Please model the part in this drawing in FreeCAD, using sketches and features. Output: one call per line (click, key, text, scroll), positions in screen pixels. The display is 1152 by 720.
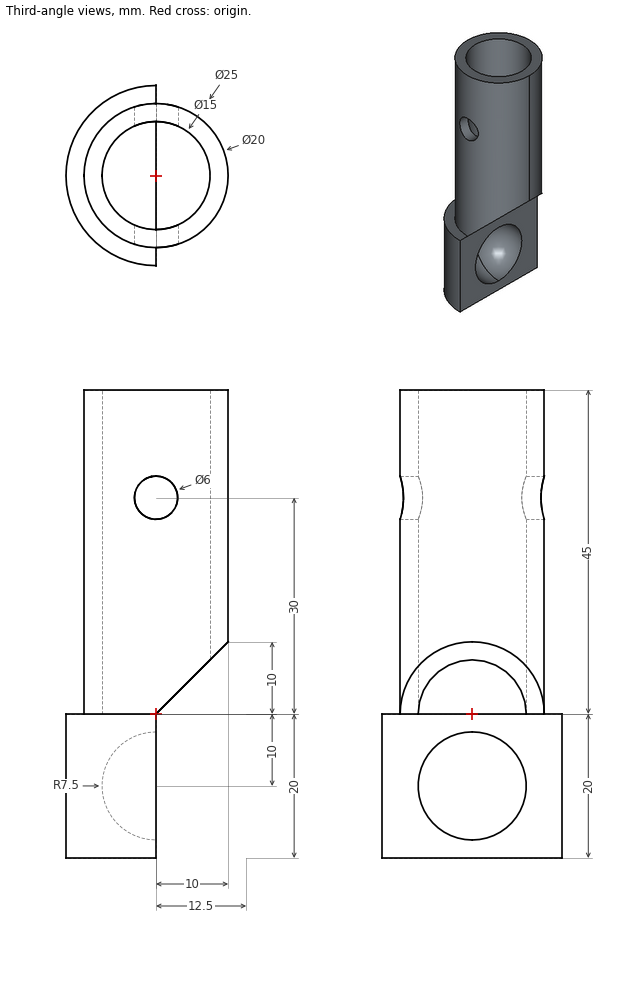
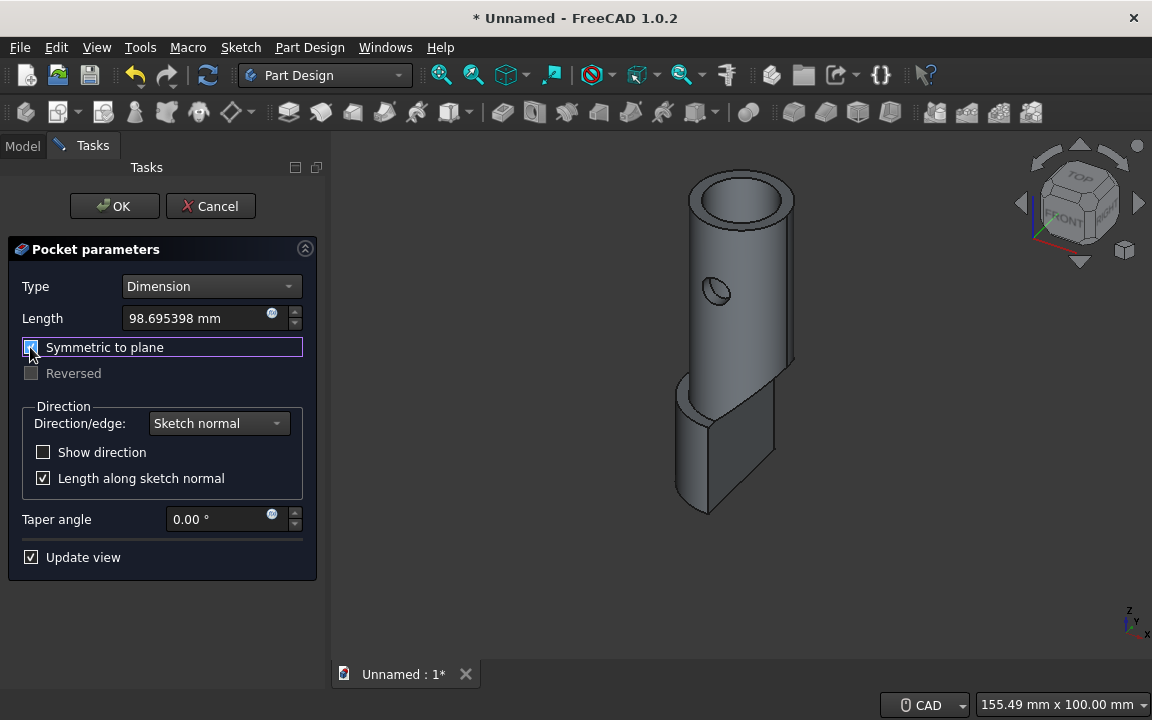
click(115, 206)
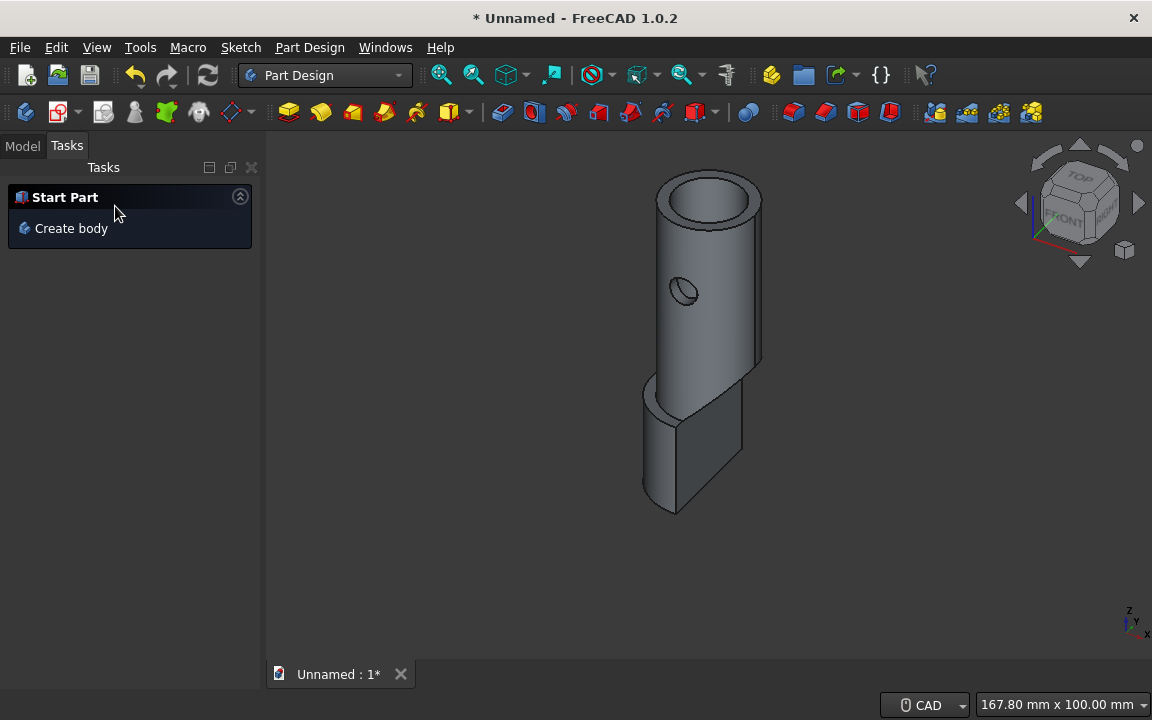
click(58, 112)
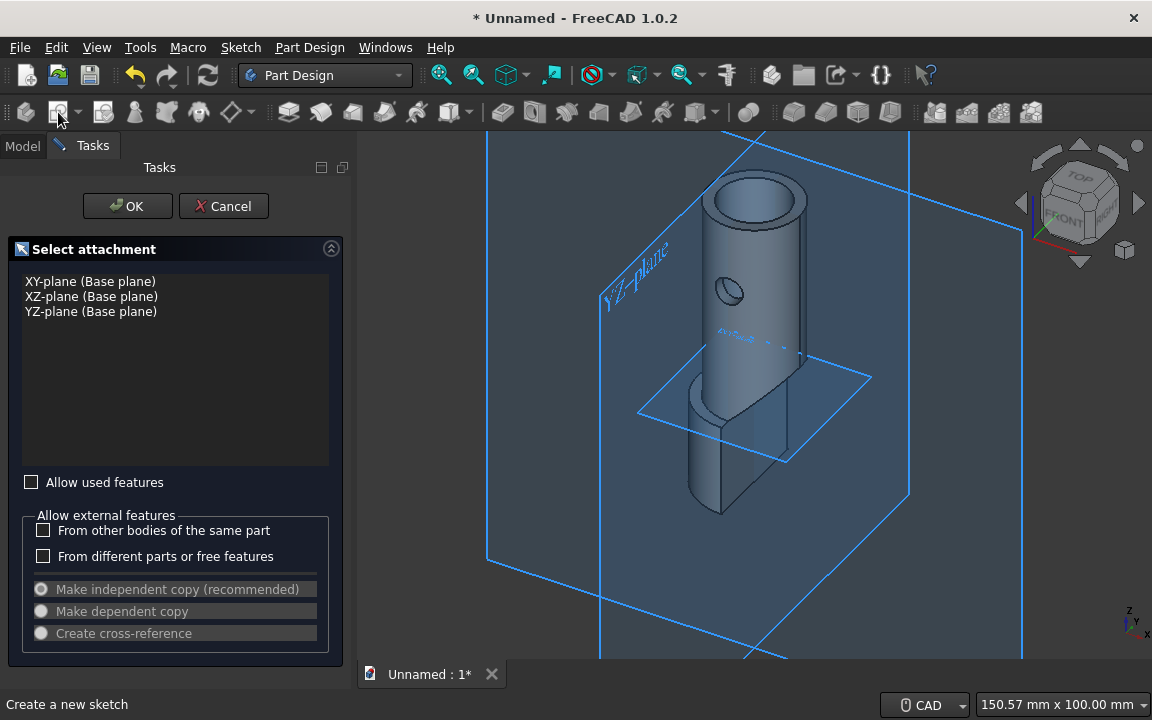
click(82, 296)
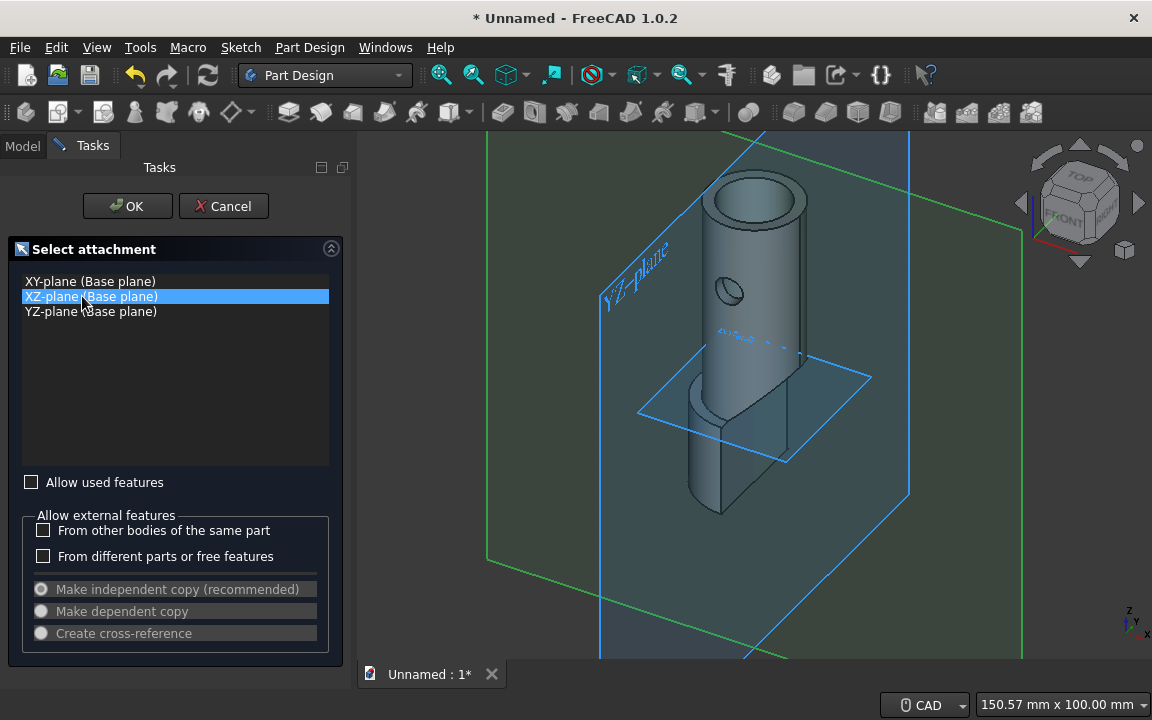
click(128, 206)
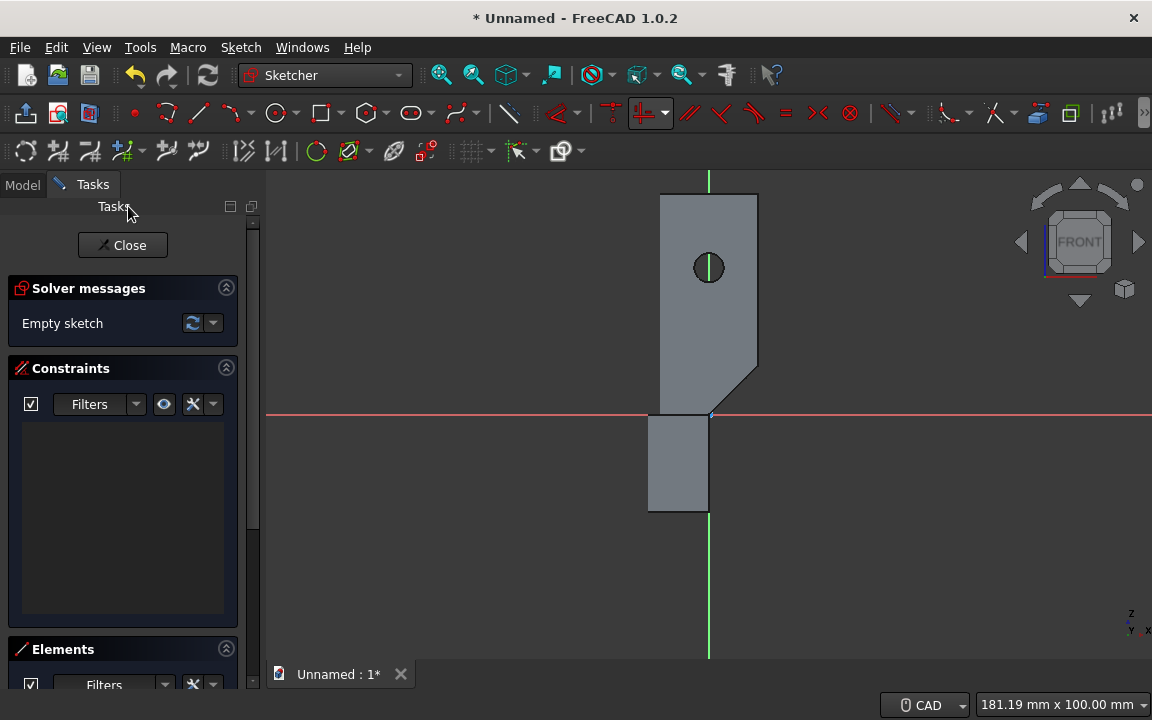
click(90, 114)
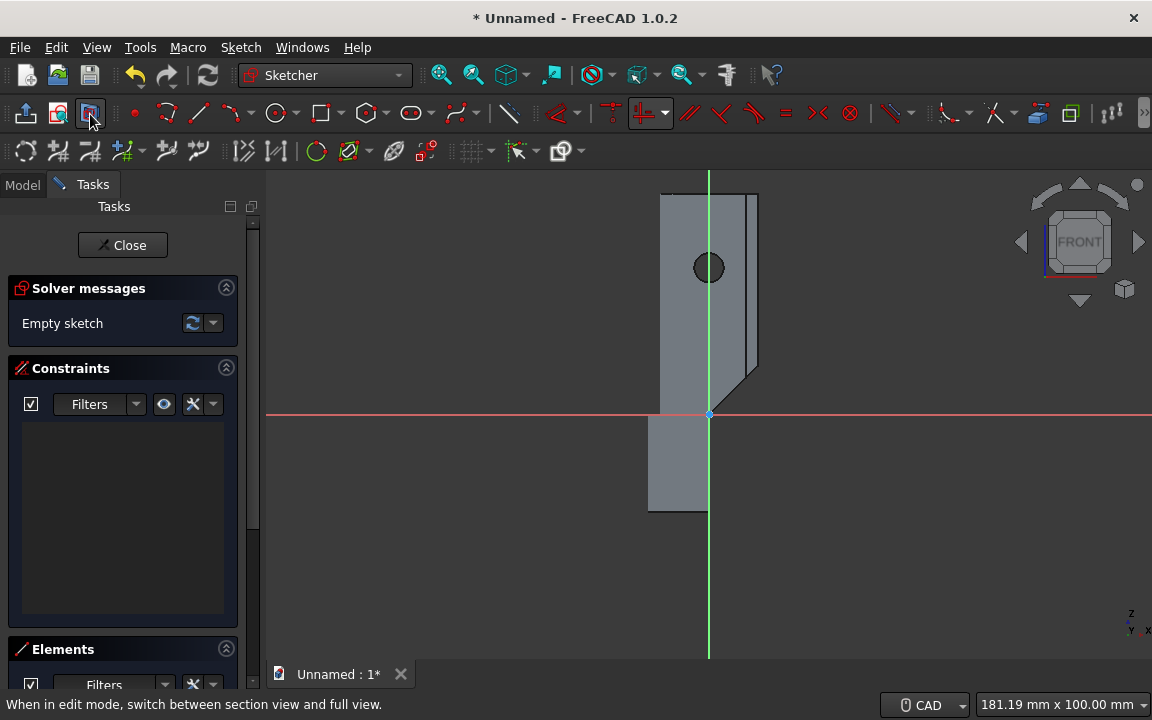
scroll(712, 476, up, 6)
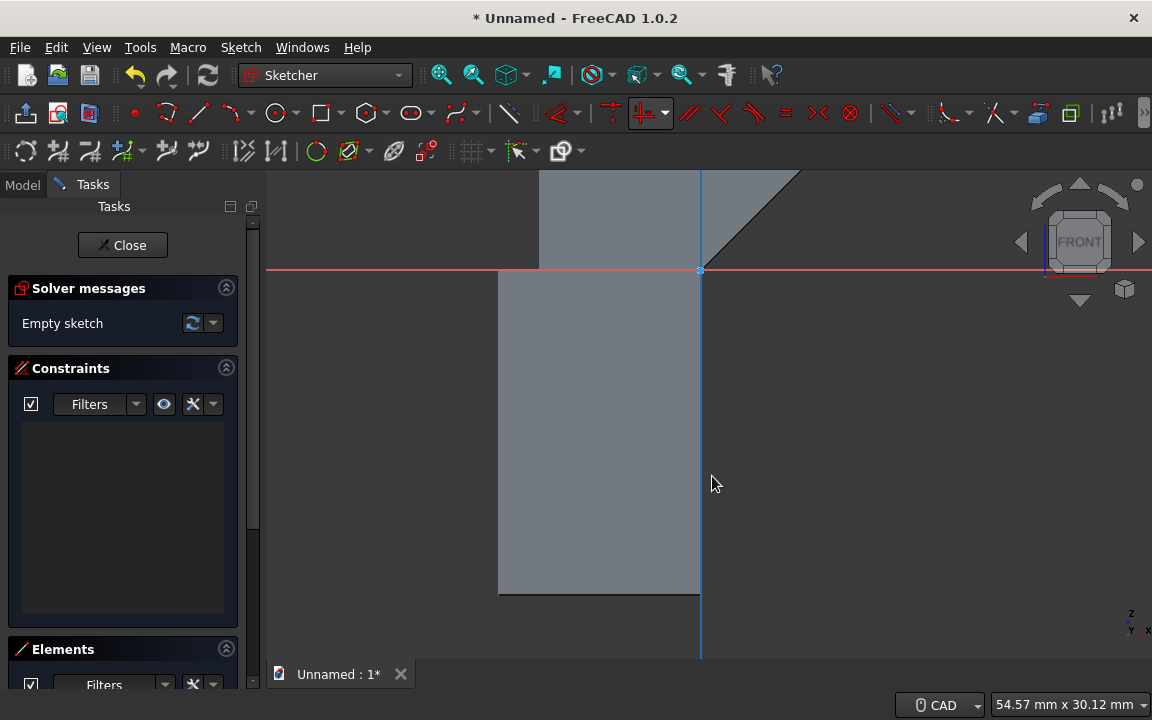
click(200, 114)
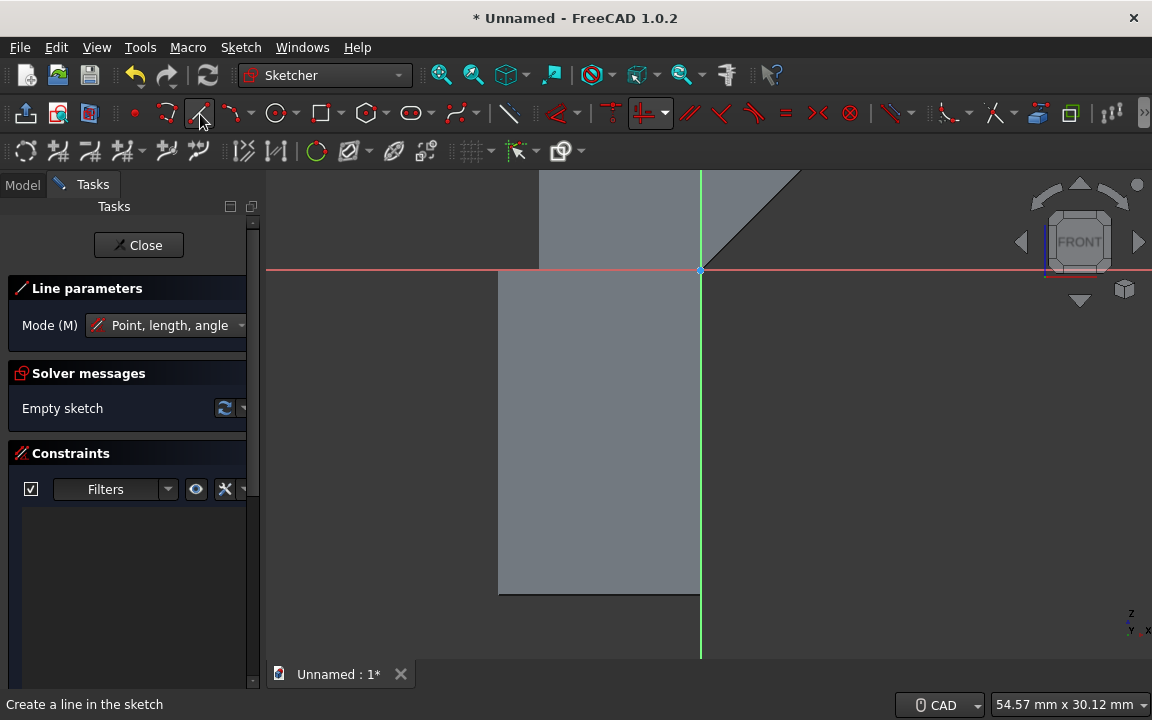
click(701, 311)
click(692, 554)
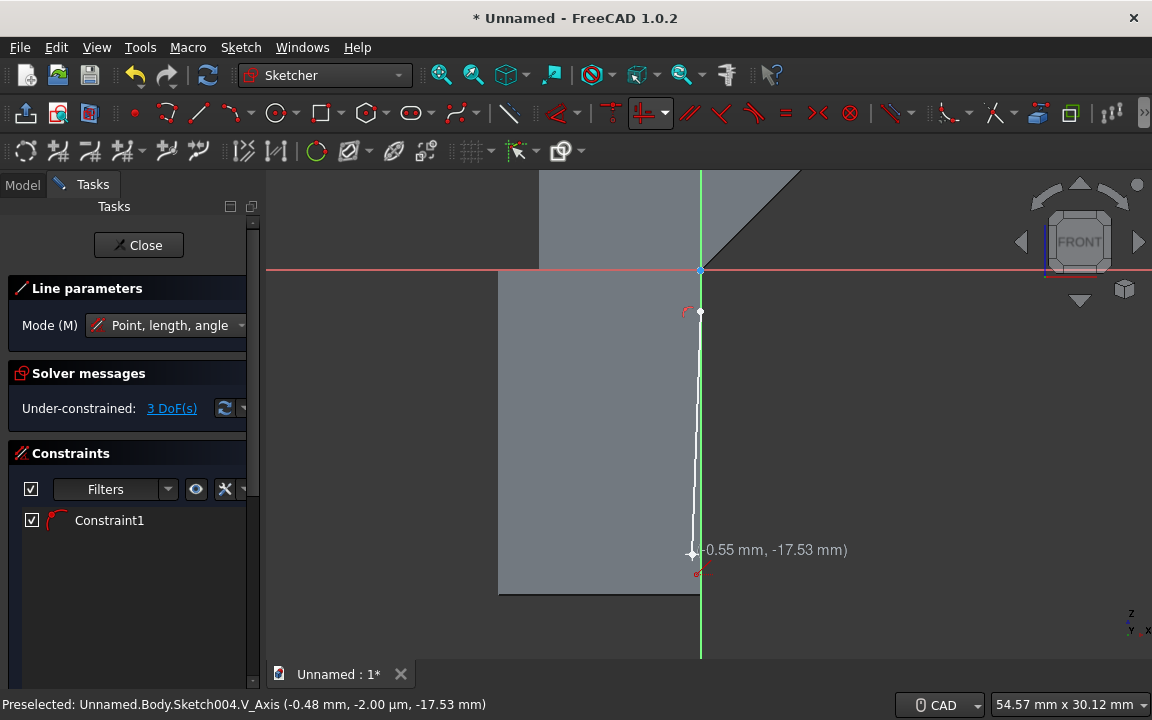
click(232, 114)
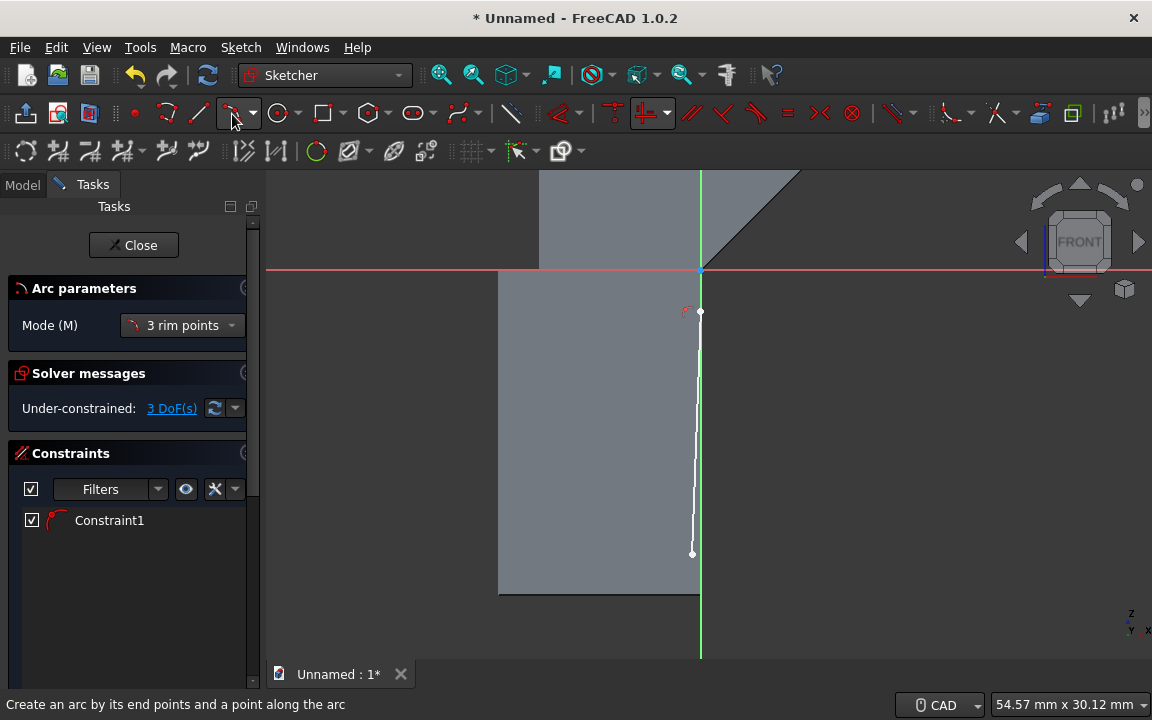
click(692, 555)
click(701, 312)
click(579, 433)
key(Escape)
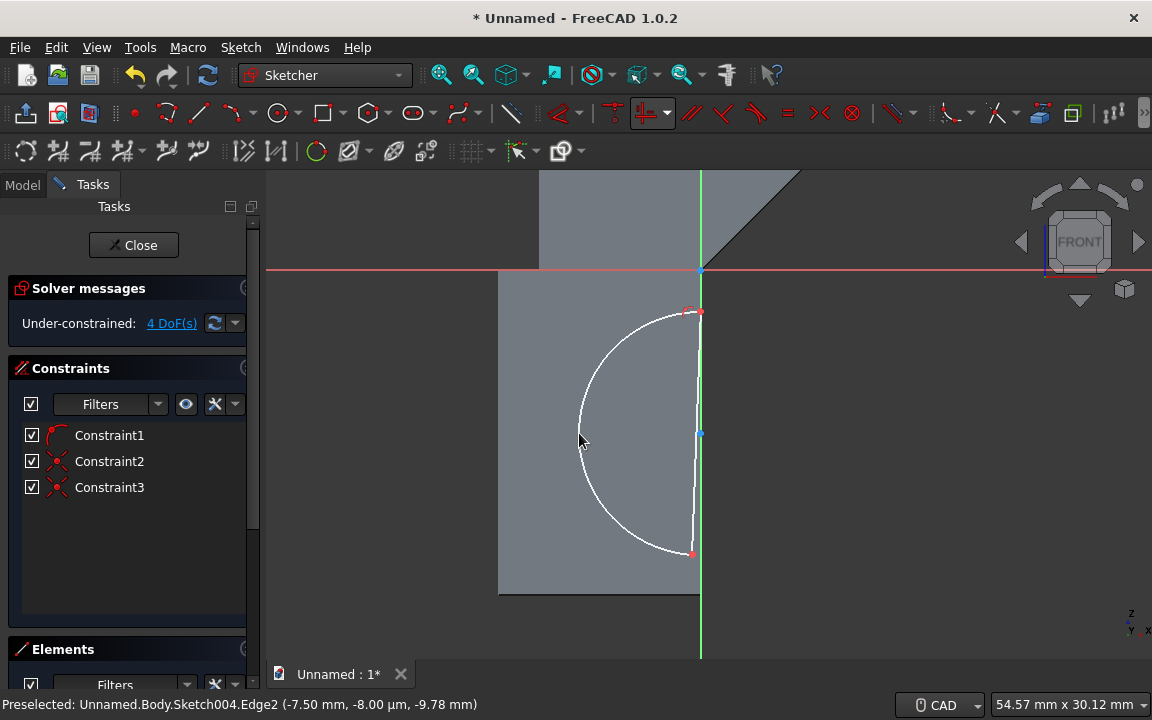
click(698, 385)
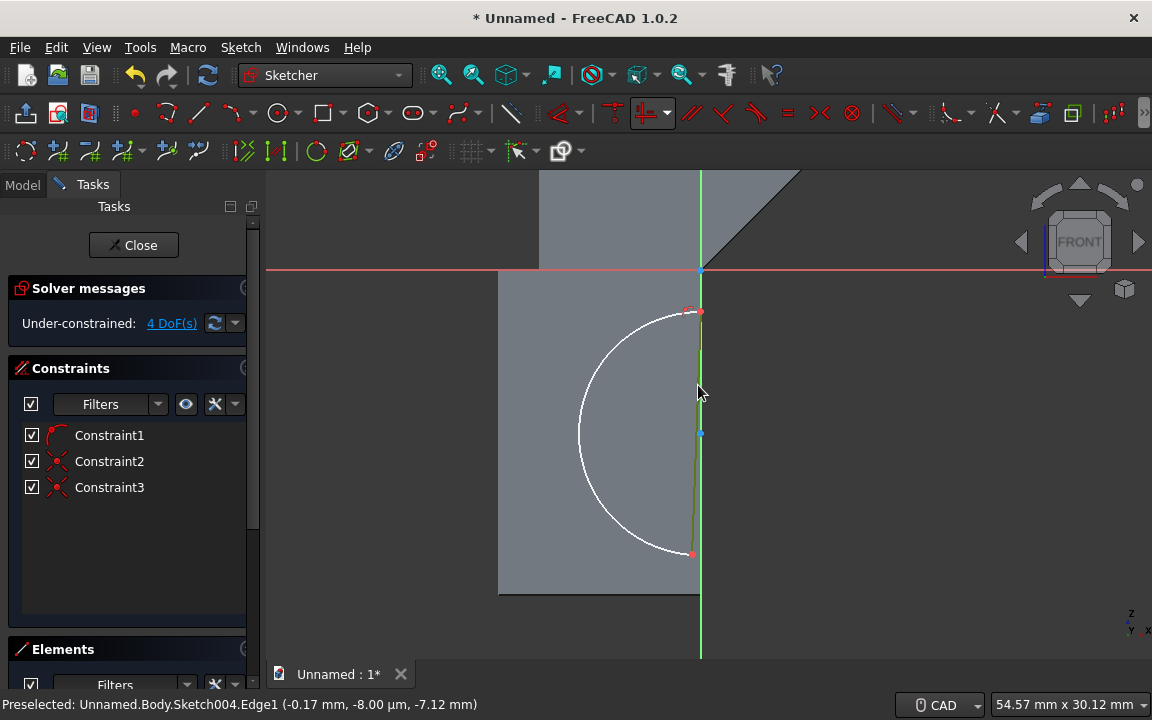
click(670, 114)